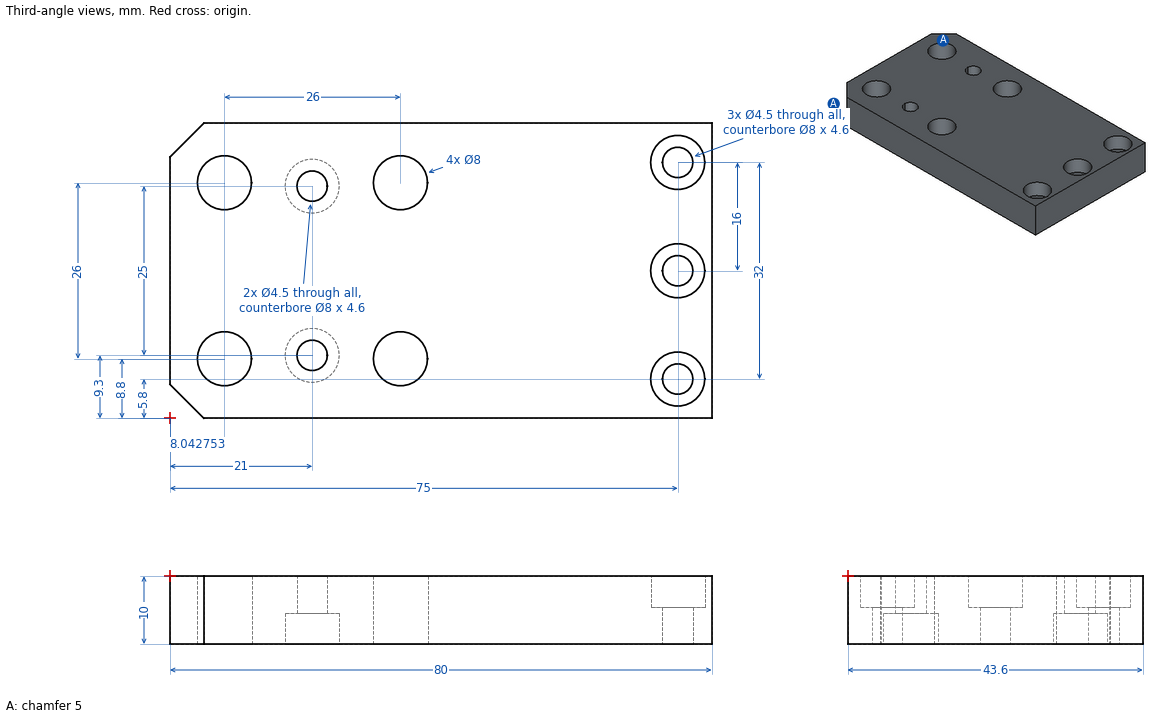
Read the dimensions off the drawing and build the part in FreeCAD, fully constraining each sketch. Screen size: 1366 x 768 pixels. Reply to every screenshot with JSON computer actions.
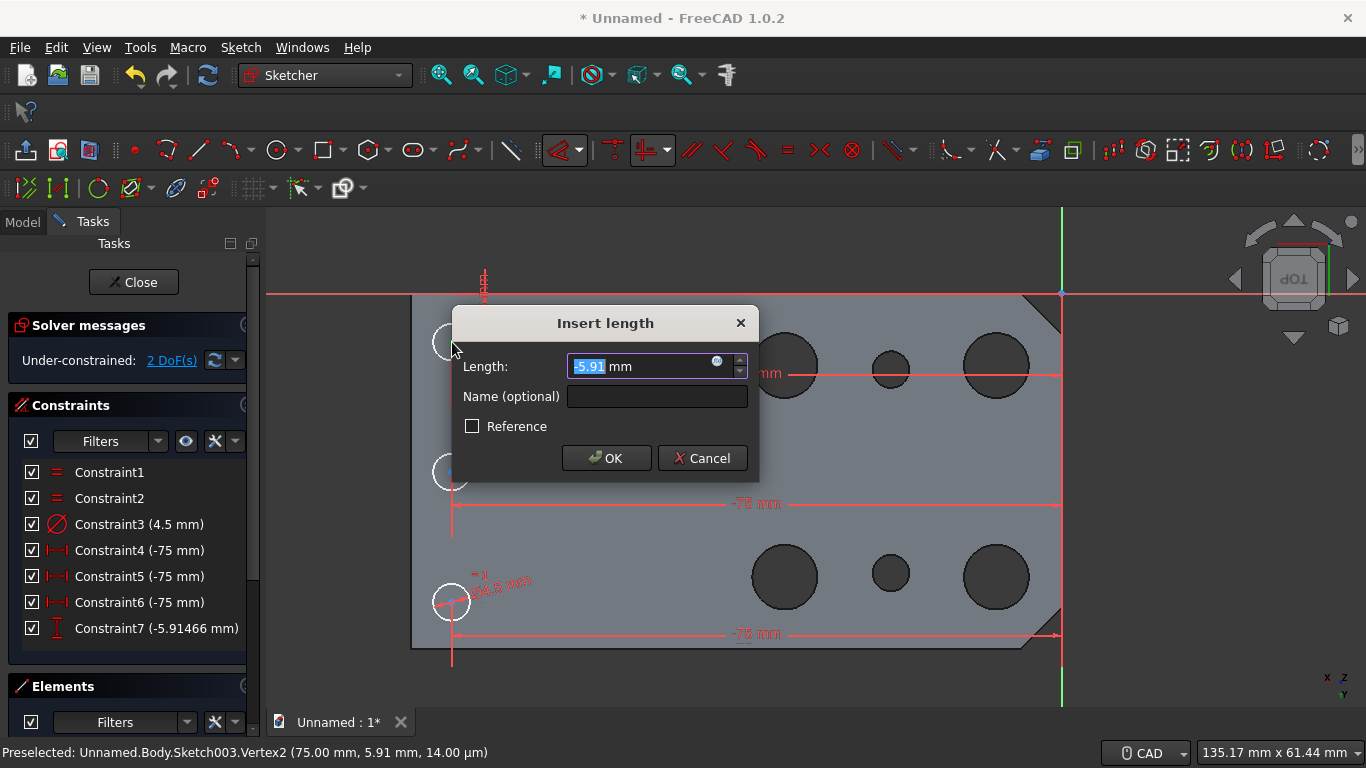
{"action": "type", "text": "-5.8"}
{"action": "key", "text": "Return"}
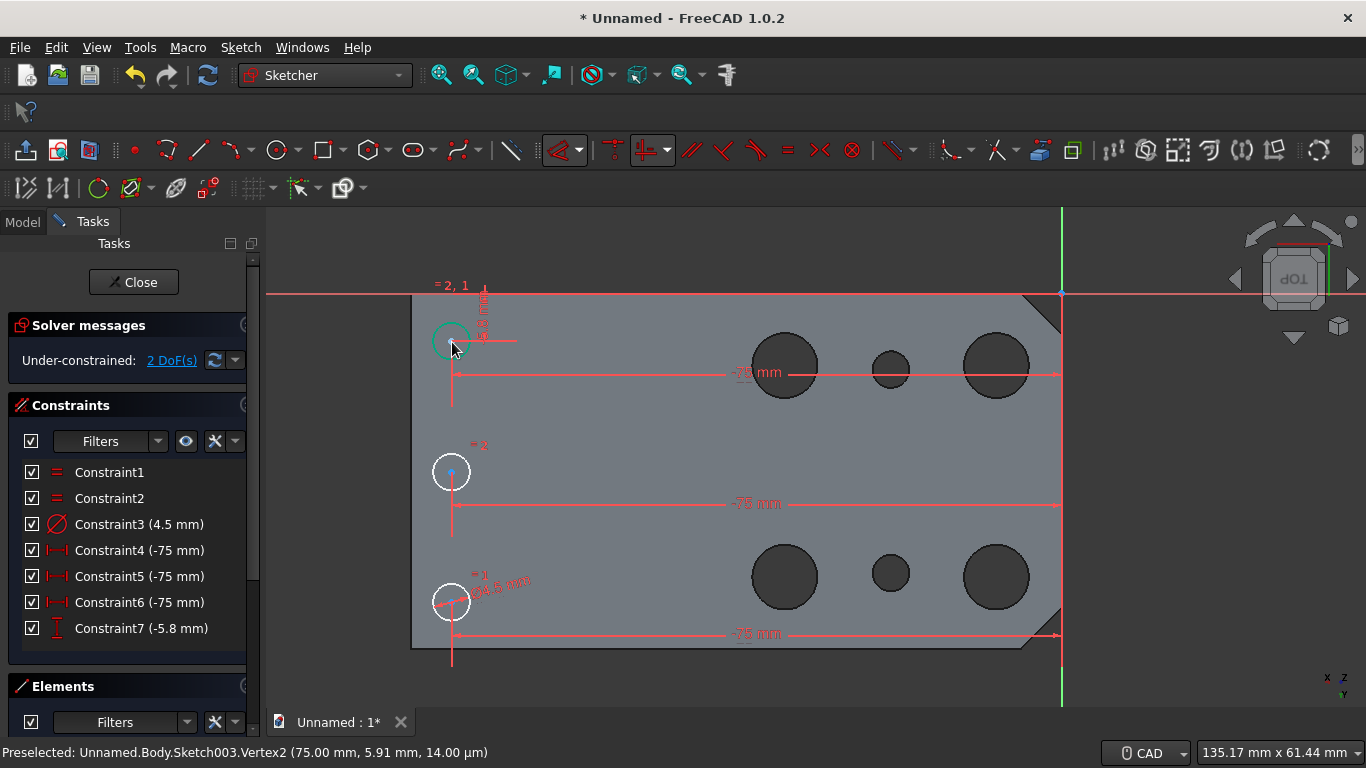
{"action": "left_click", "coordinate": [452, 602]}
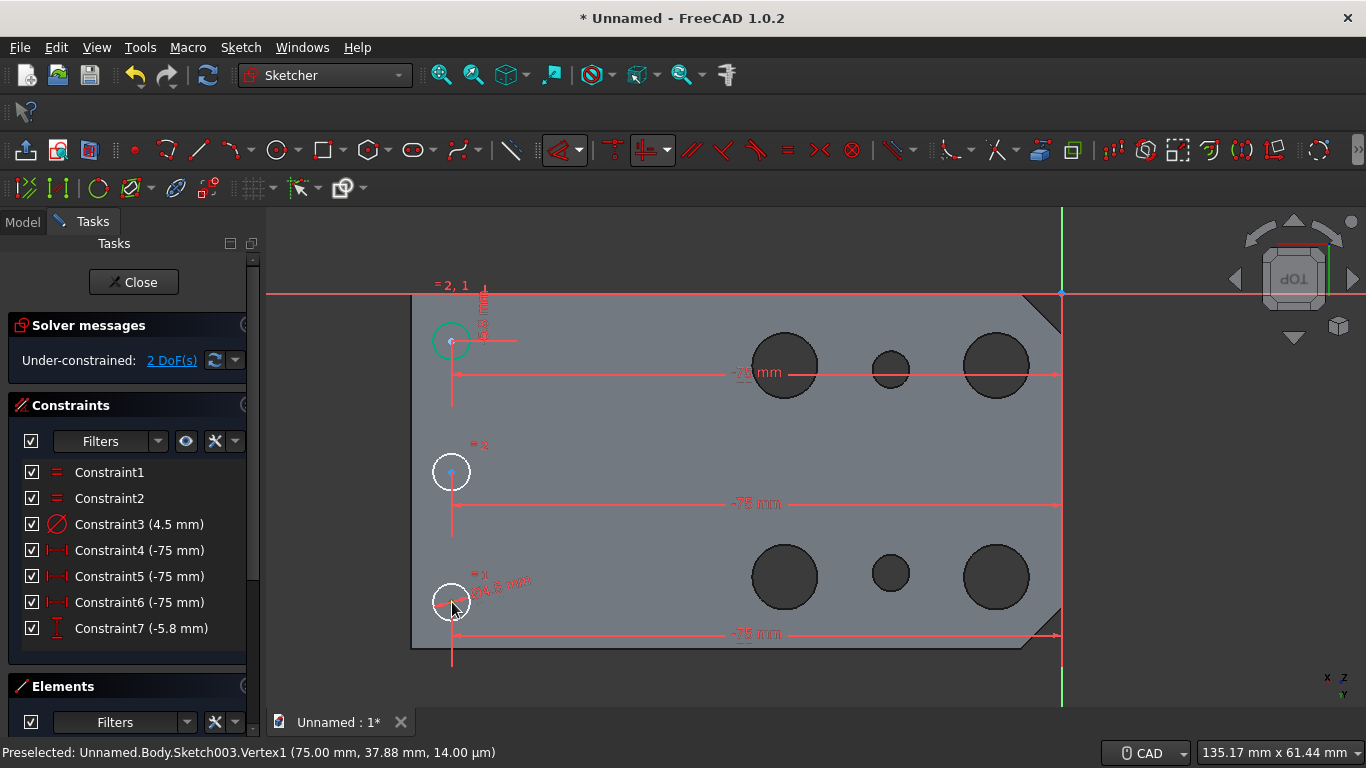
{"action": "left_click", "coordinate": [452, 341]}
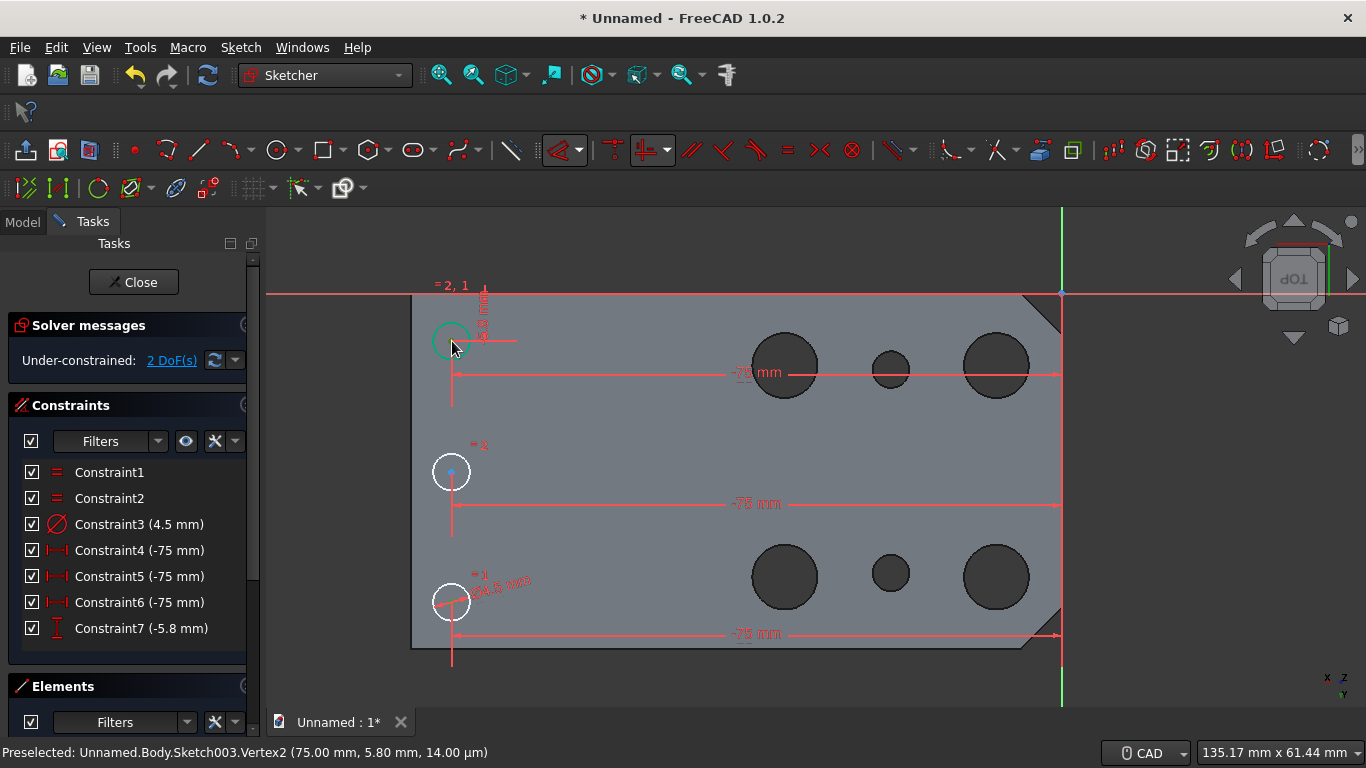
{"action": "left_click", "coordinate": [582, 150]}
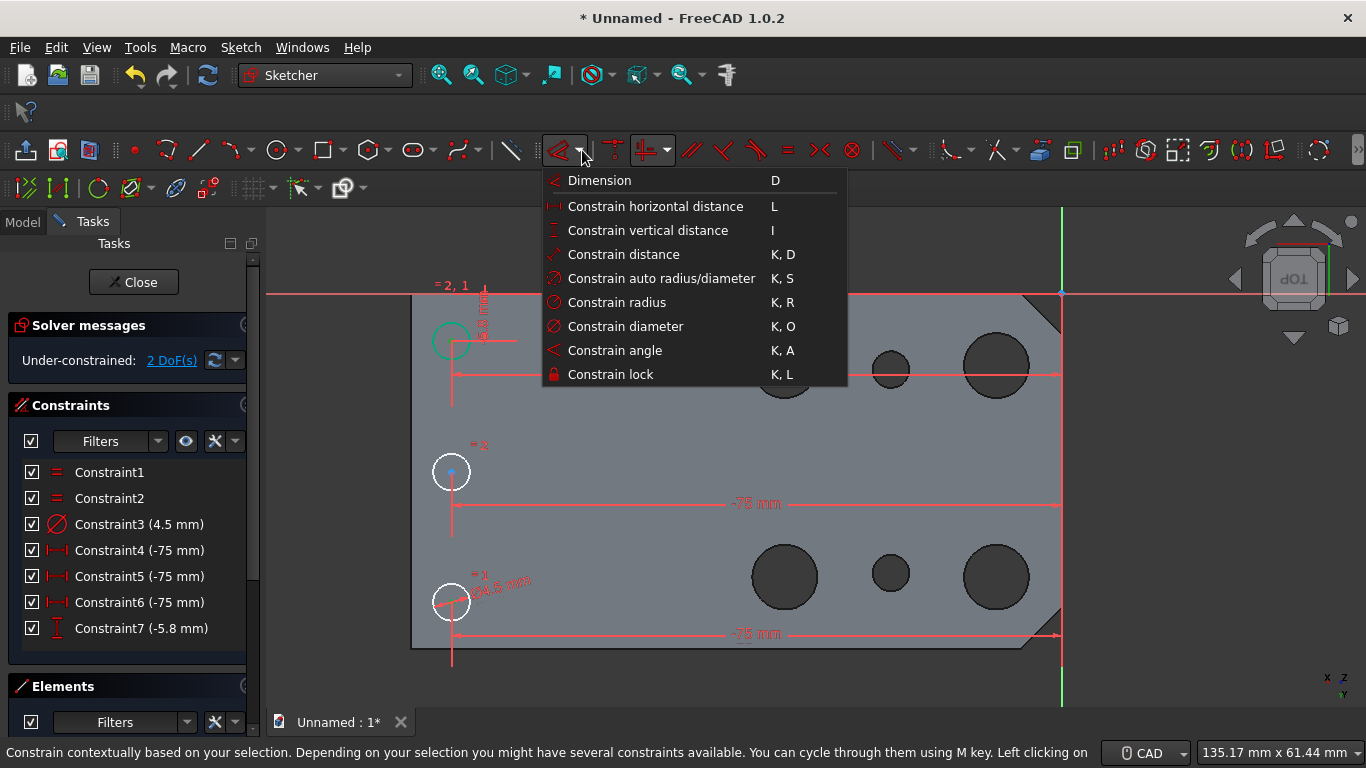
{"action": "left_click", "coordinate": [695, 230]}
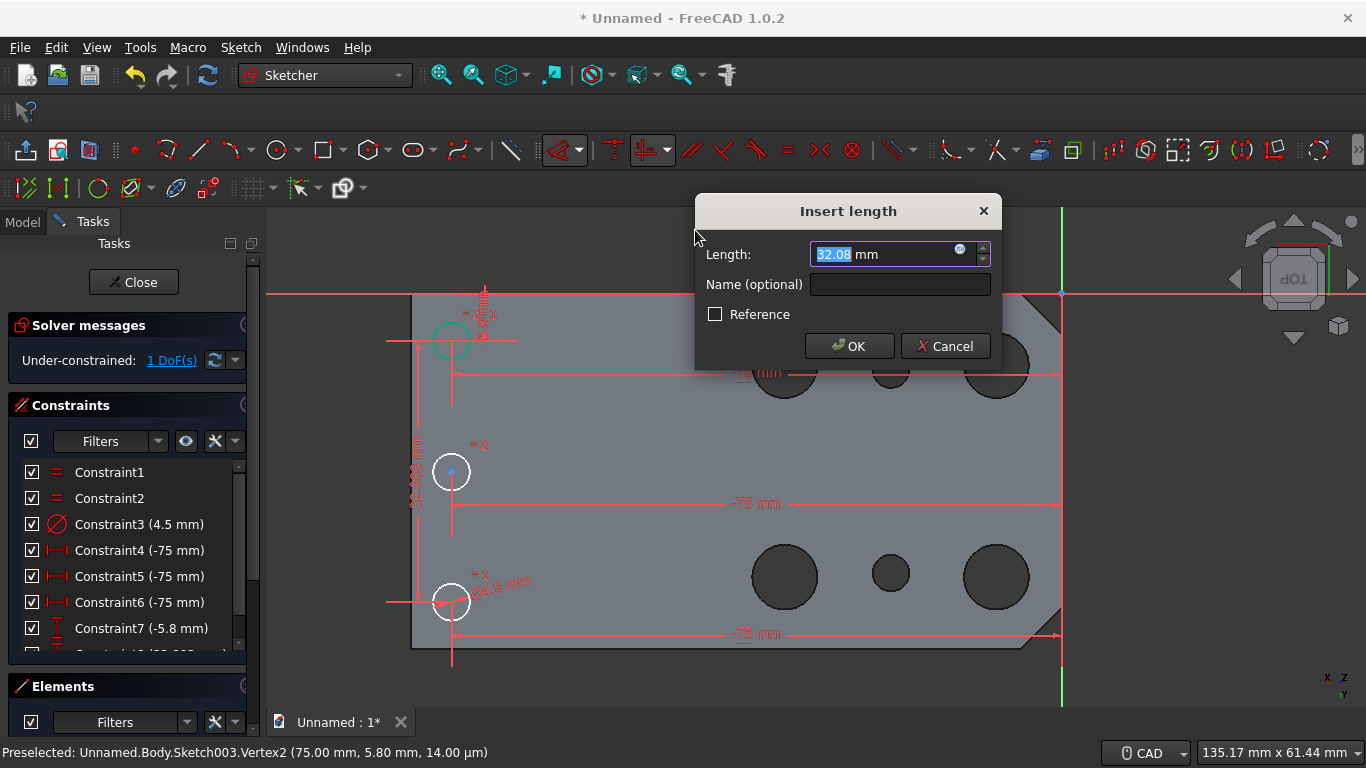
{"action": "type", "text": "32"}
{"action": "key", "text": "Return"}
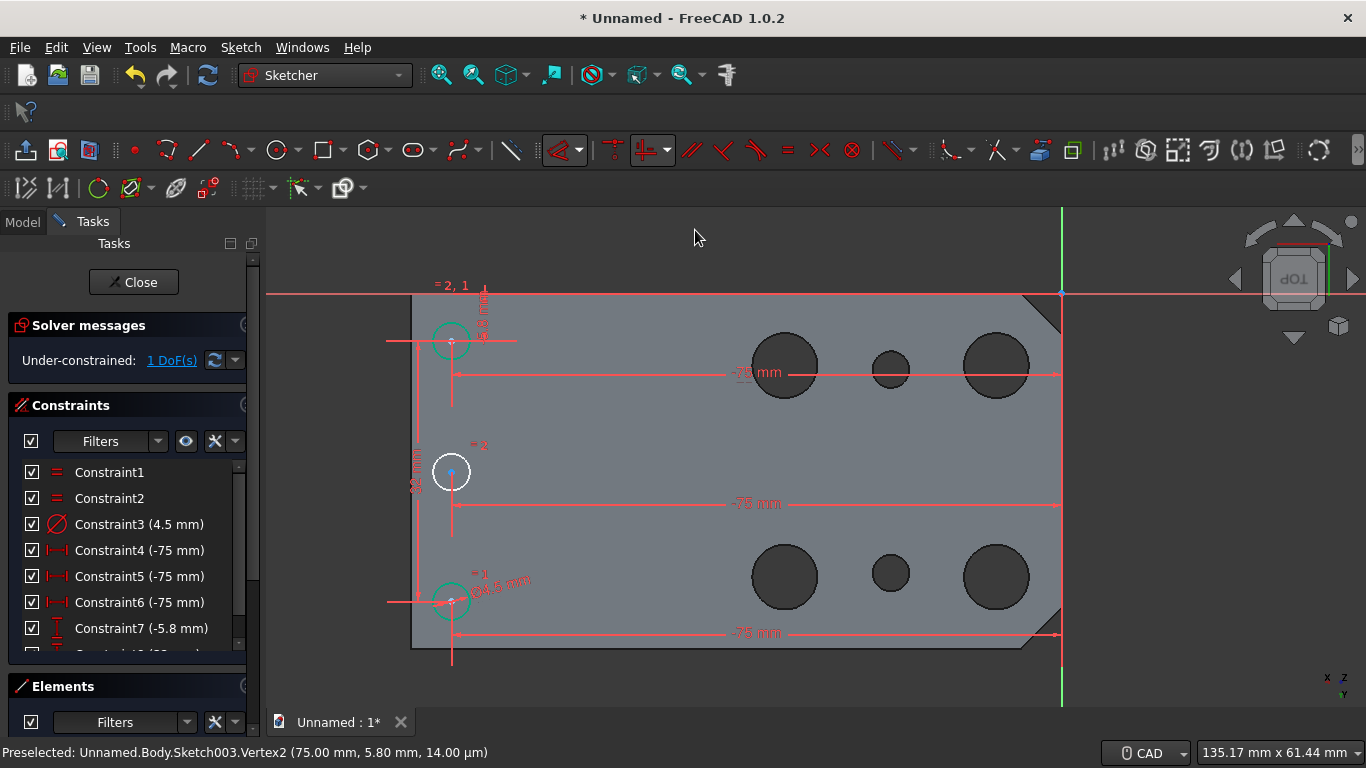
{"action": "left_click", "coordinate": [452, 602]}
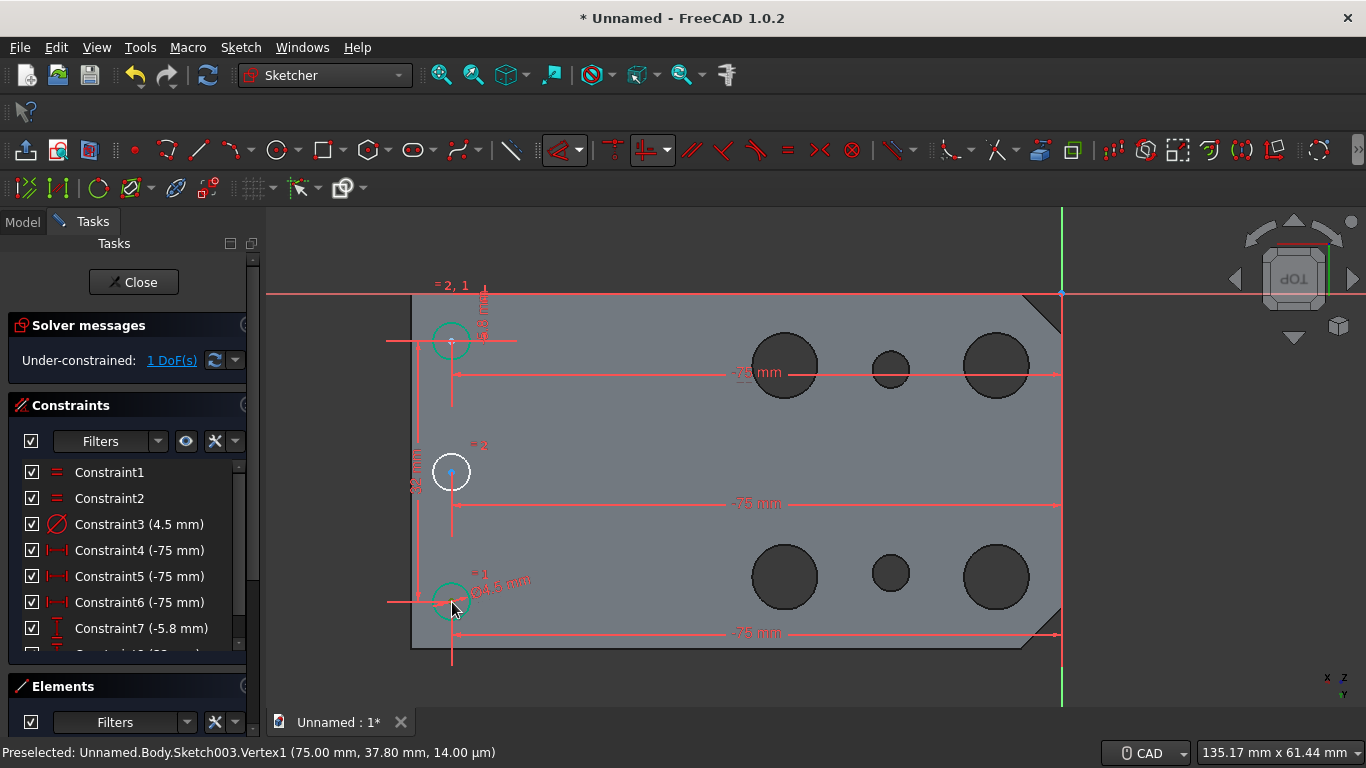
{"action": "left_click", "coordinate": [452, 472]}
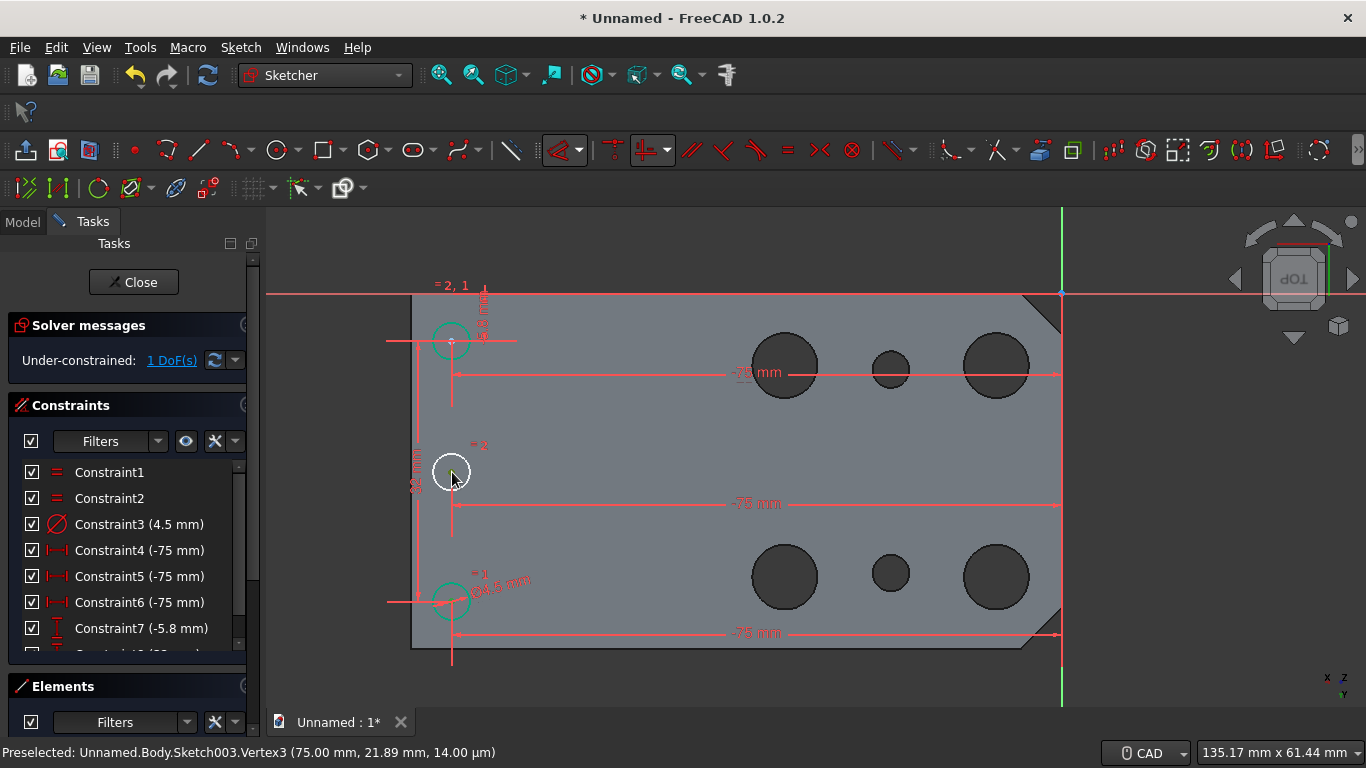
{"action": "key", "text": "i"}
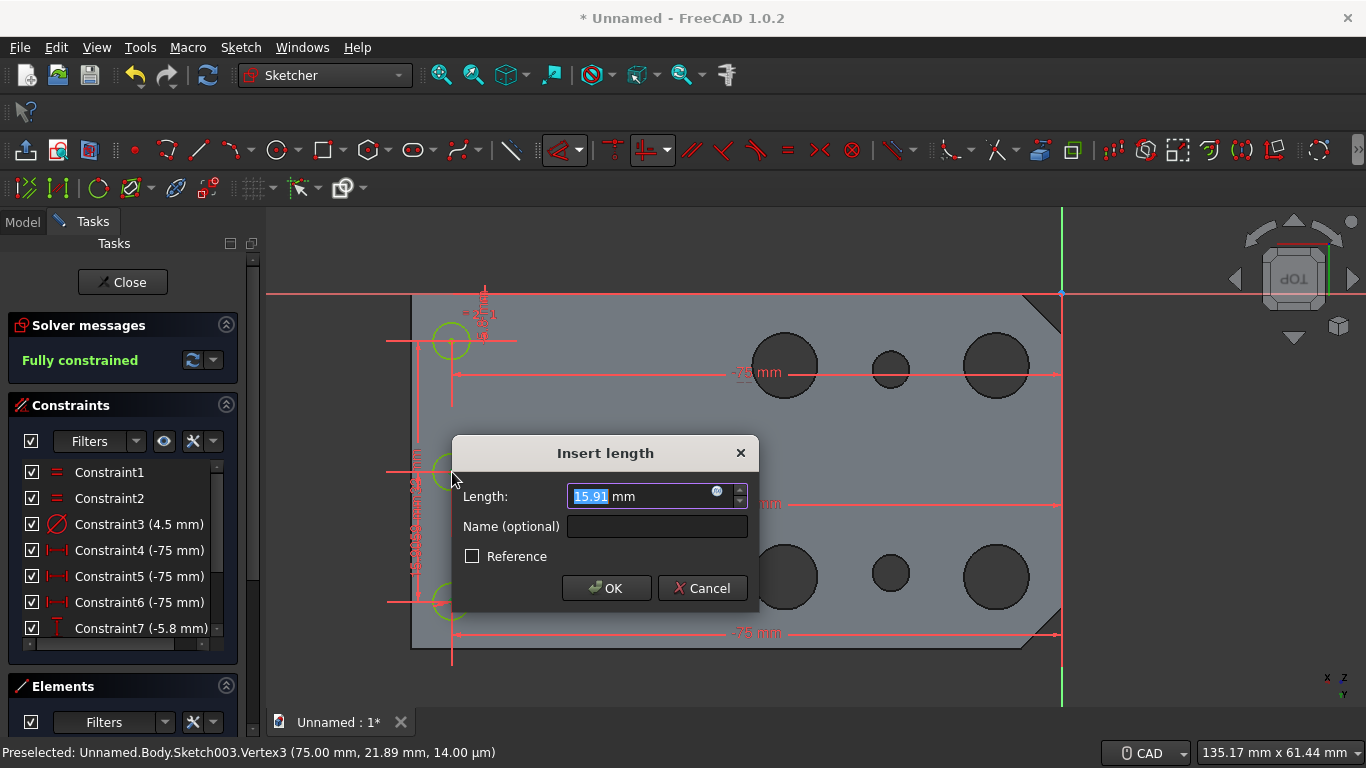
{"action": "type", "text": "16"}
{"action": "key", "text": "Return"}